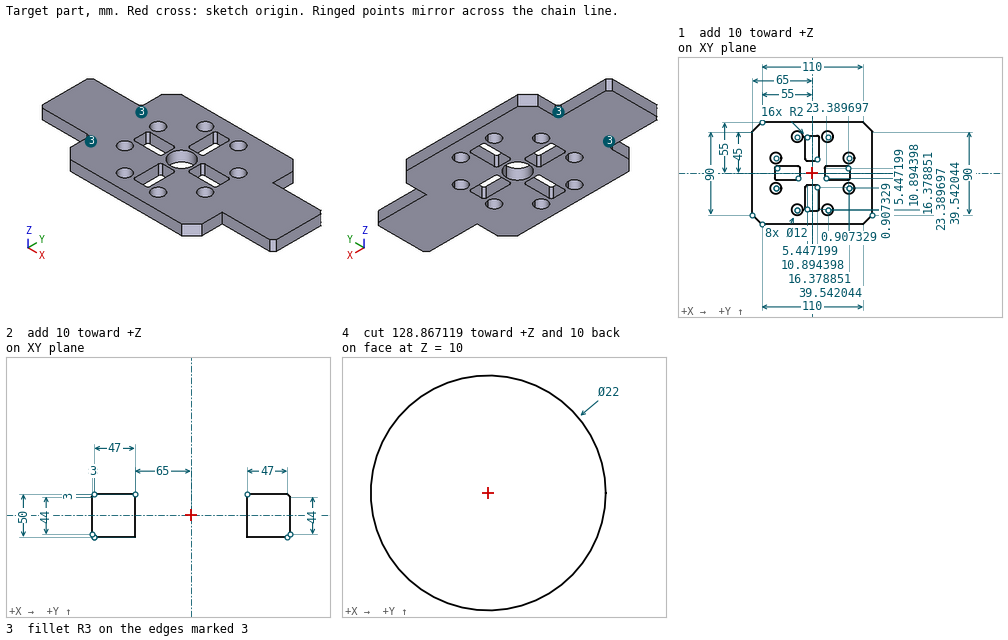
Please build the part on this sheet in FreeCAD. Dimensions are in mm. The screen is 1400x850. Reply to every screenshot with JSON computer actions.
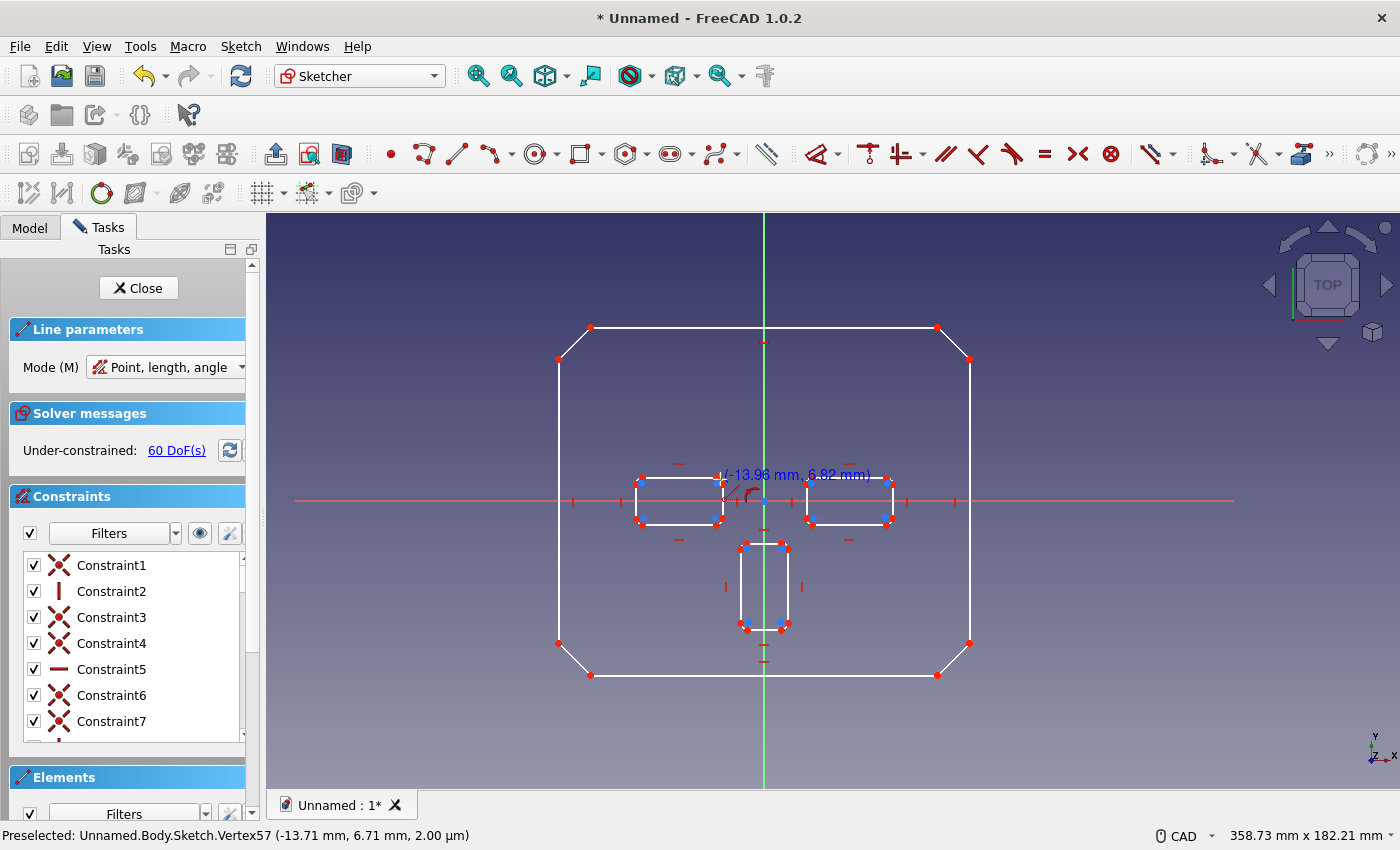
{"action": "left_click", "coordinate": [788, 379]}
{"action": "left_click", "coordinate": [788, 453]}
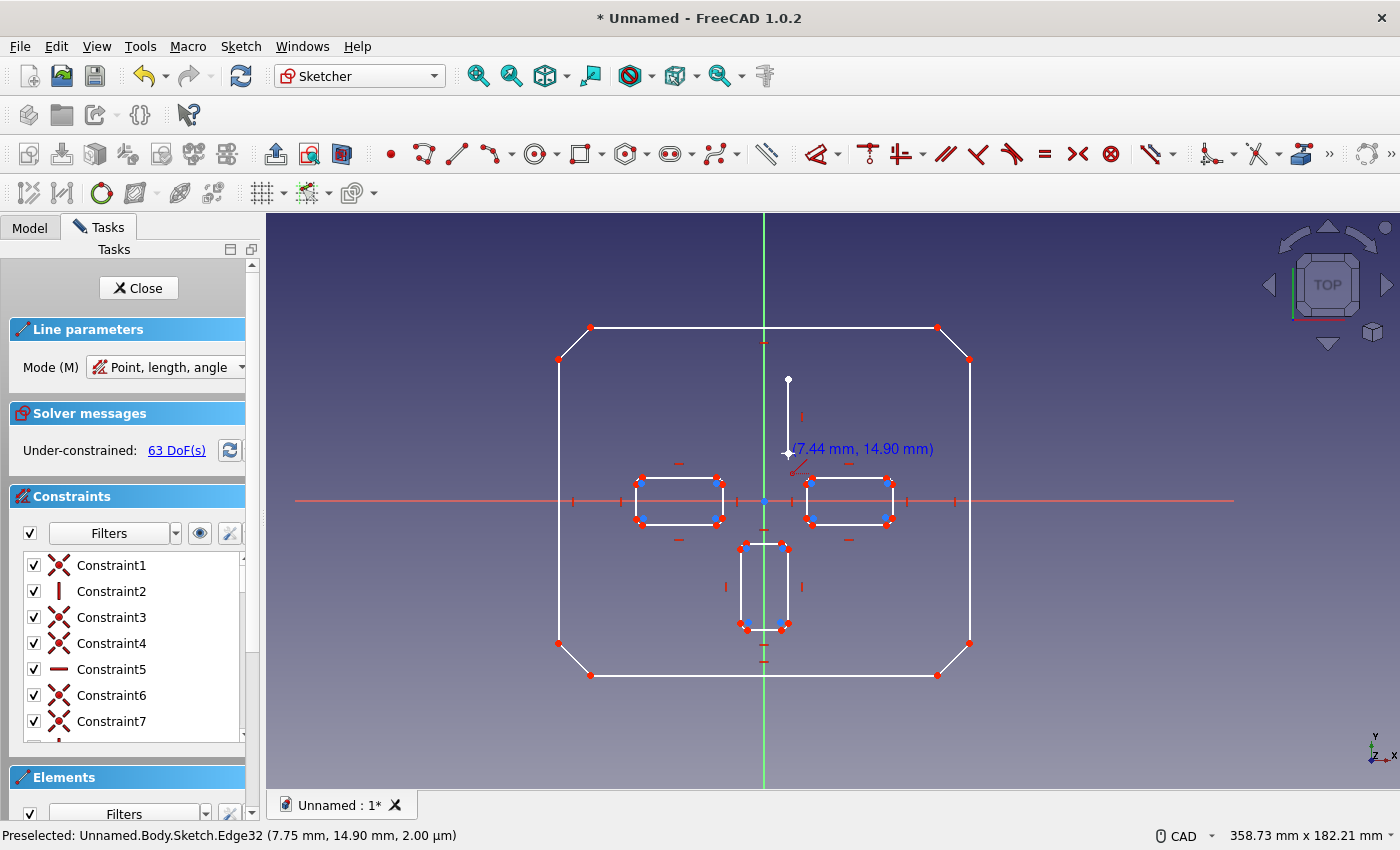
{"action": "scroll", "coordinate": [782, 459], "scroll_direction": "up", "scroll_amount": 3}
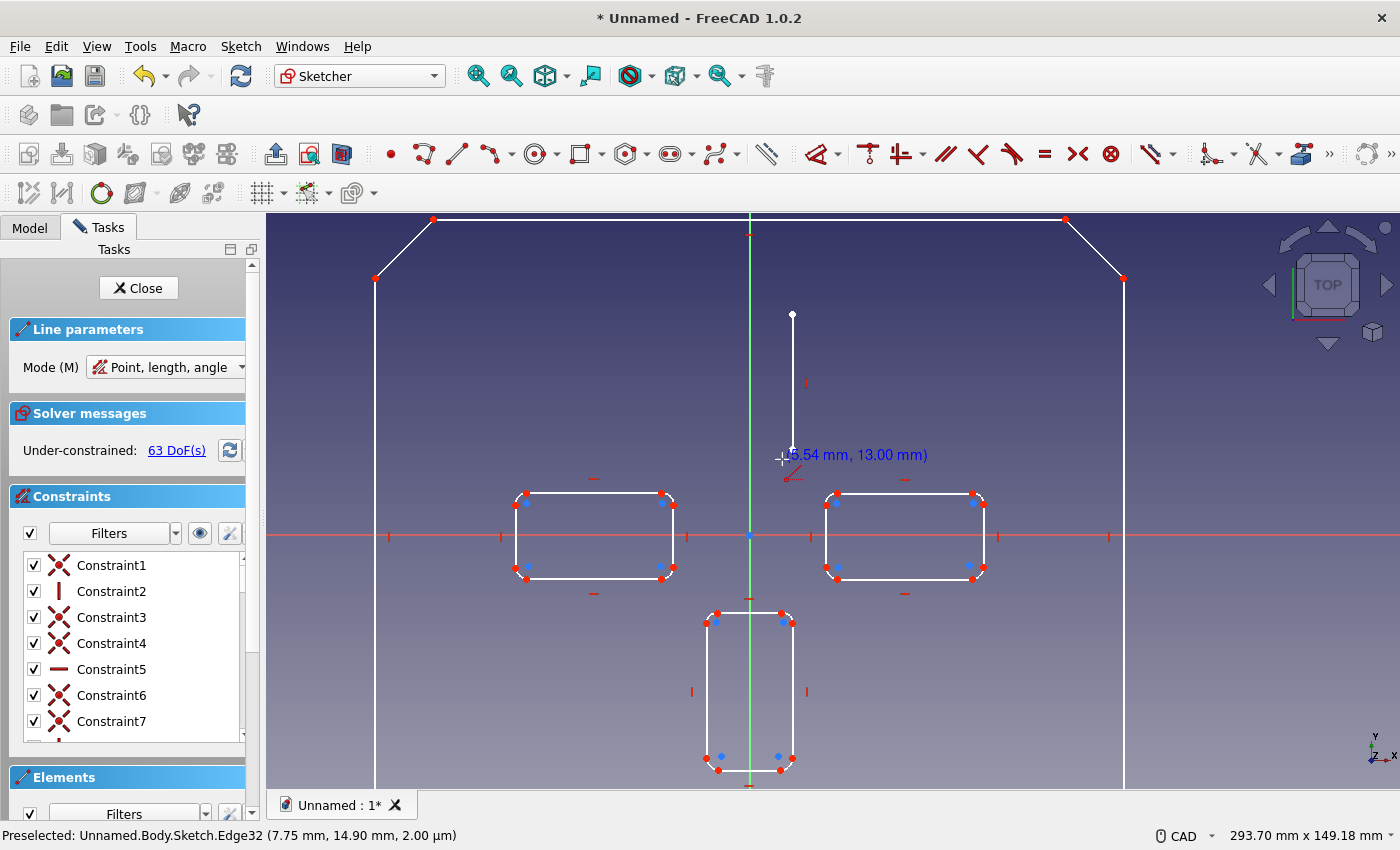
{"action": "left_click", "coordinate": [781, 459]}
{"action": "left_click", "coordinate": [718, 459]}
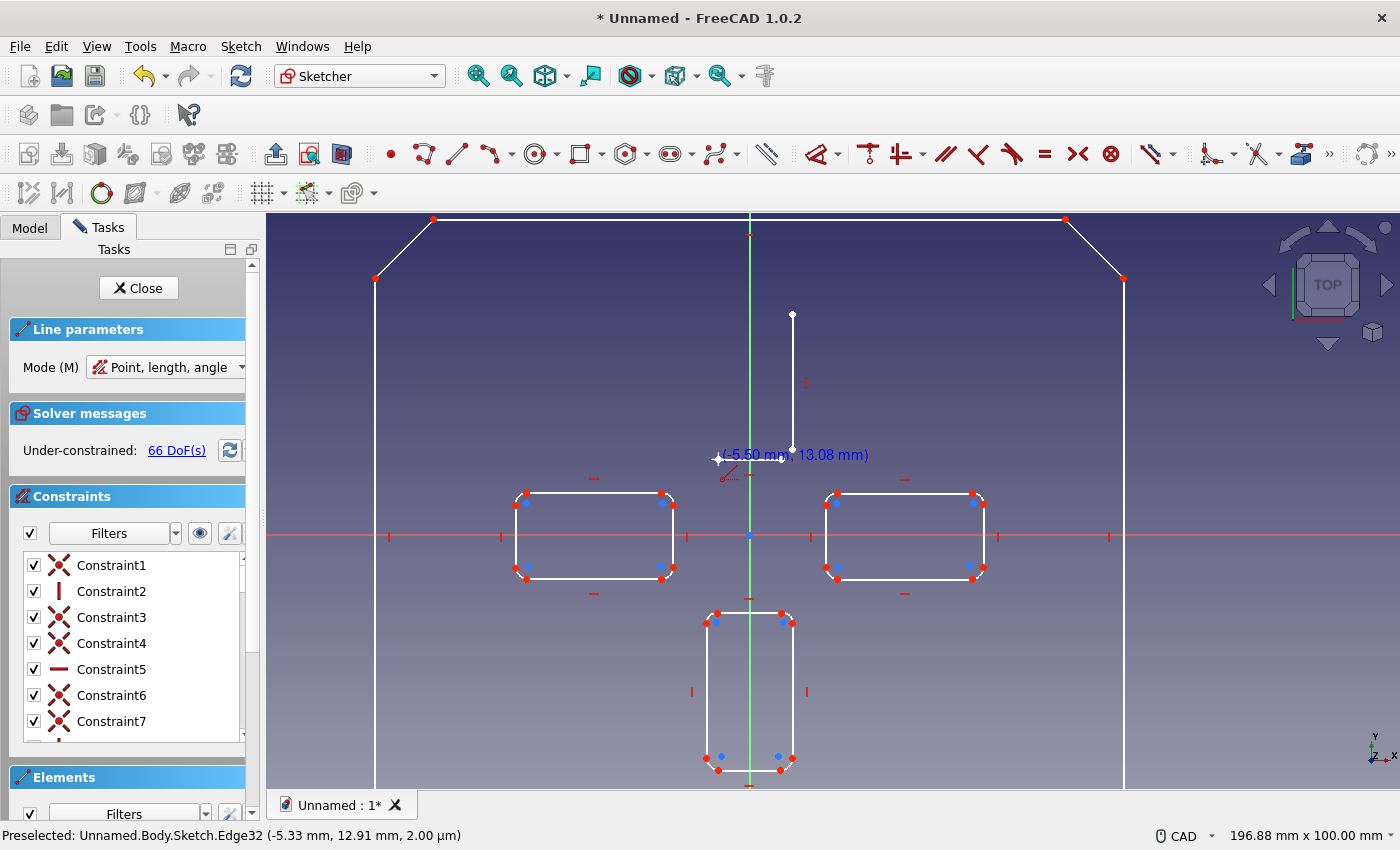
{"action": "left_click", "coordinate": [707, 448]}
{"action": "left_click", "coordinate": [707, 313]}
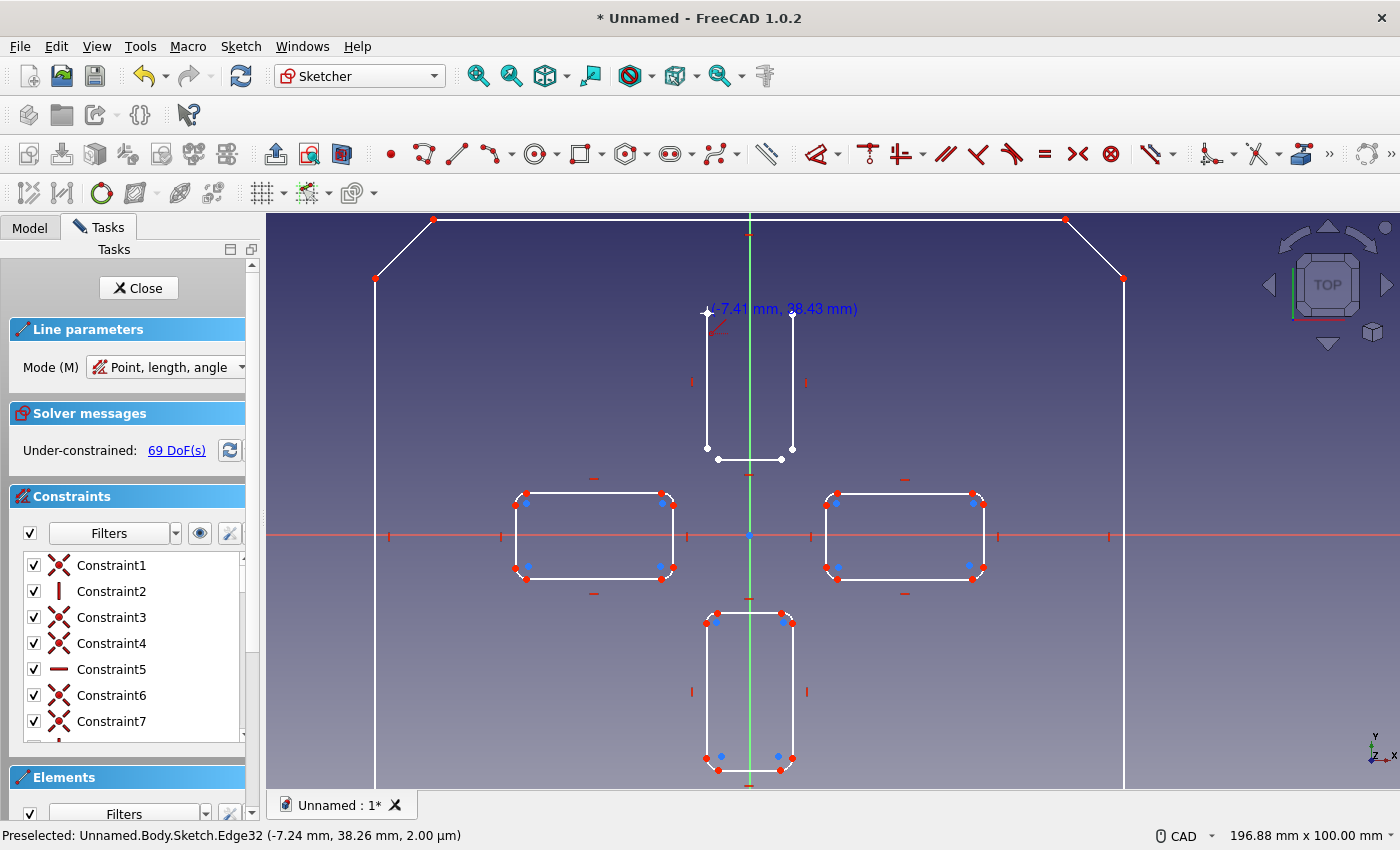
{"action": "left_click", "coordinate": [718, 301]}
{"action": "left_click", "coordinate": [781, 301]}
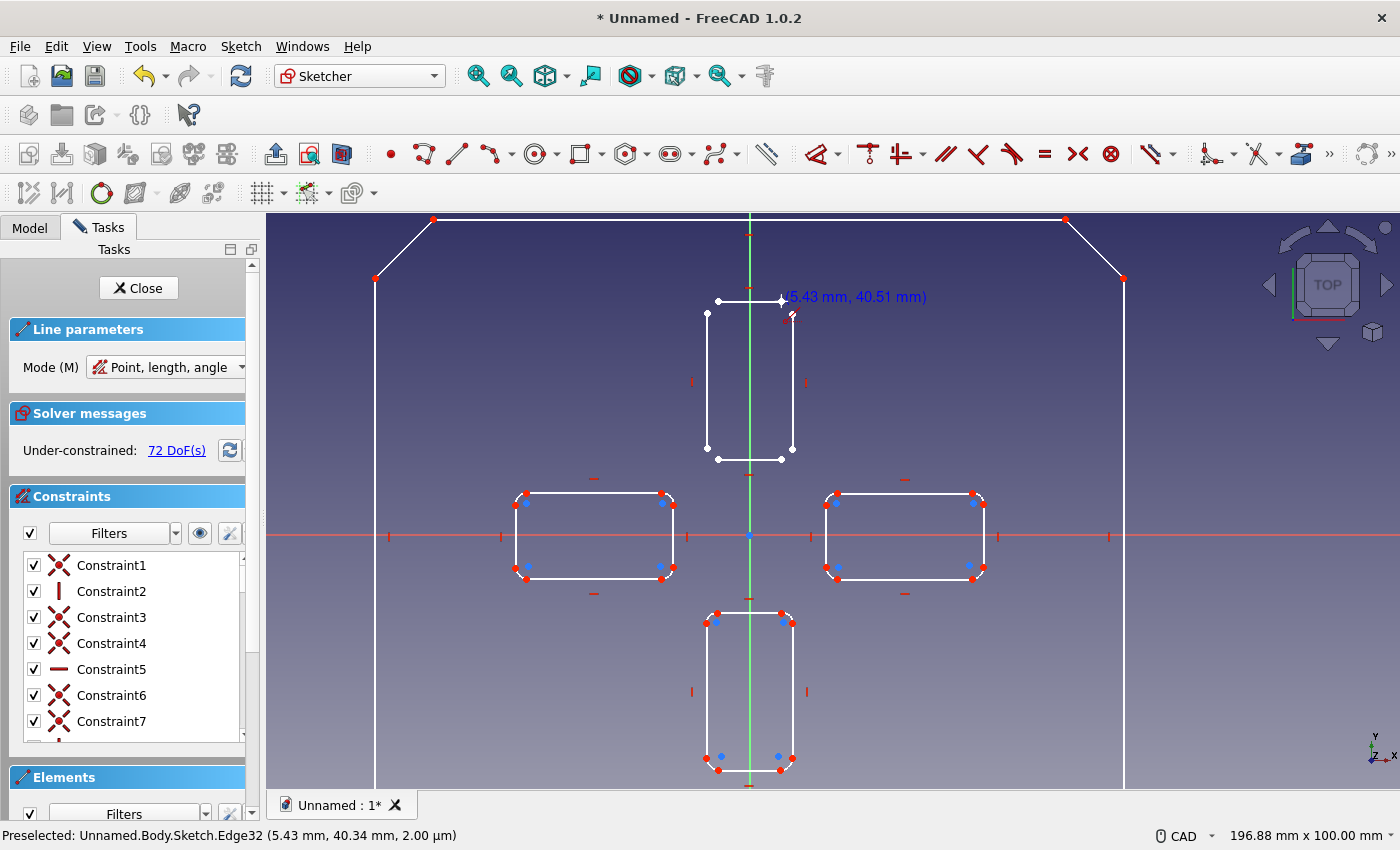
{"action": "left_click", "coordinate": [490, 154]}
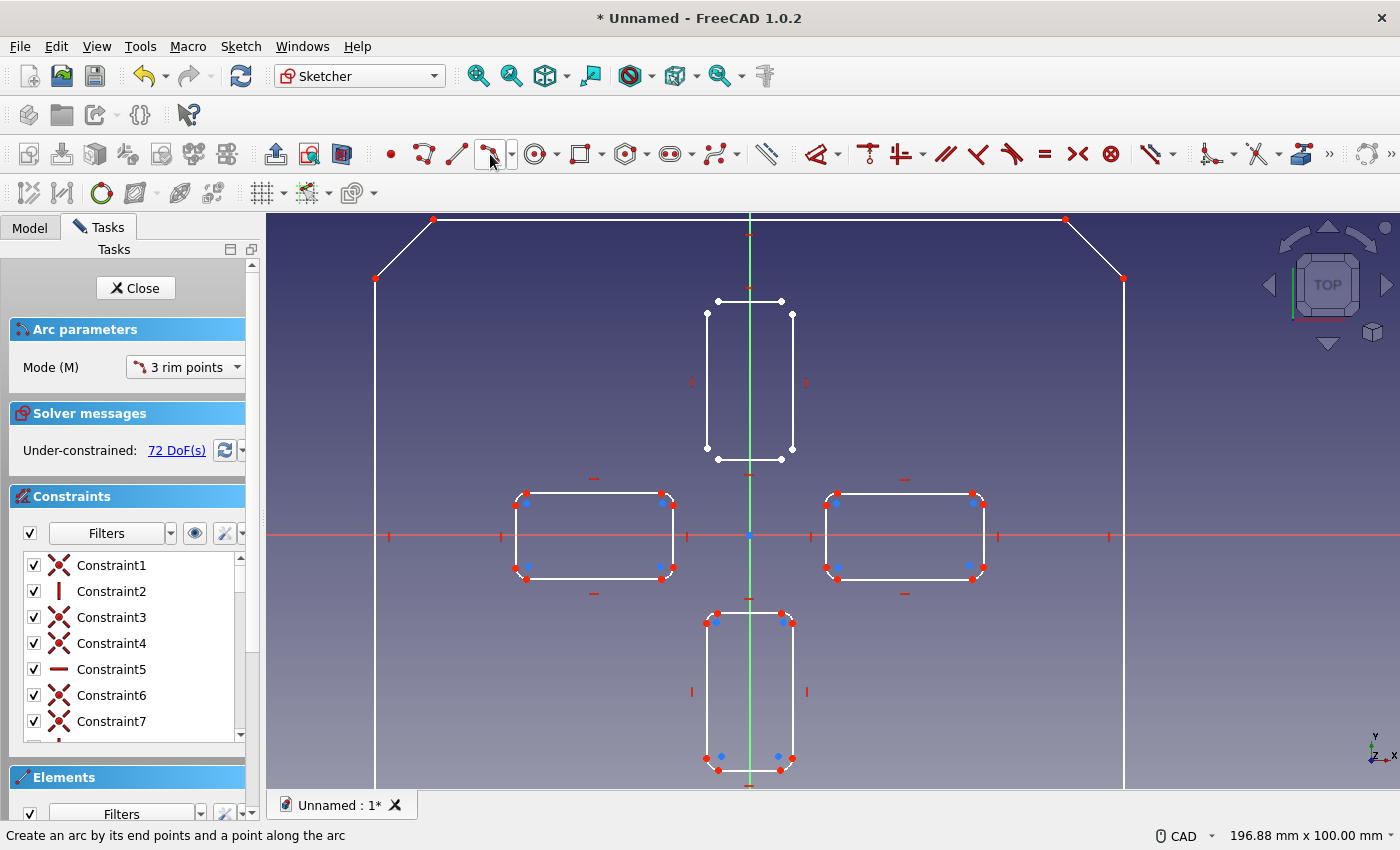
{"action": "left_click", "coordinate": [793, 450]}
{"action": "left_click", "coordinate": [781, 460]}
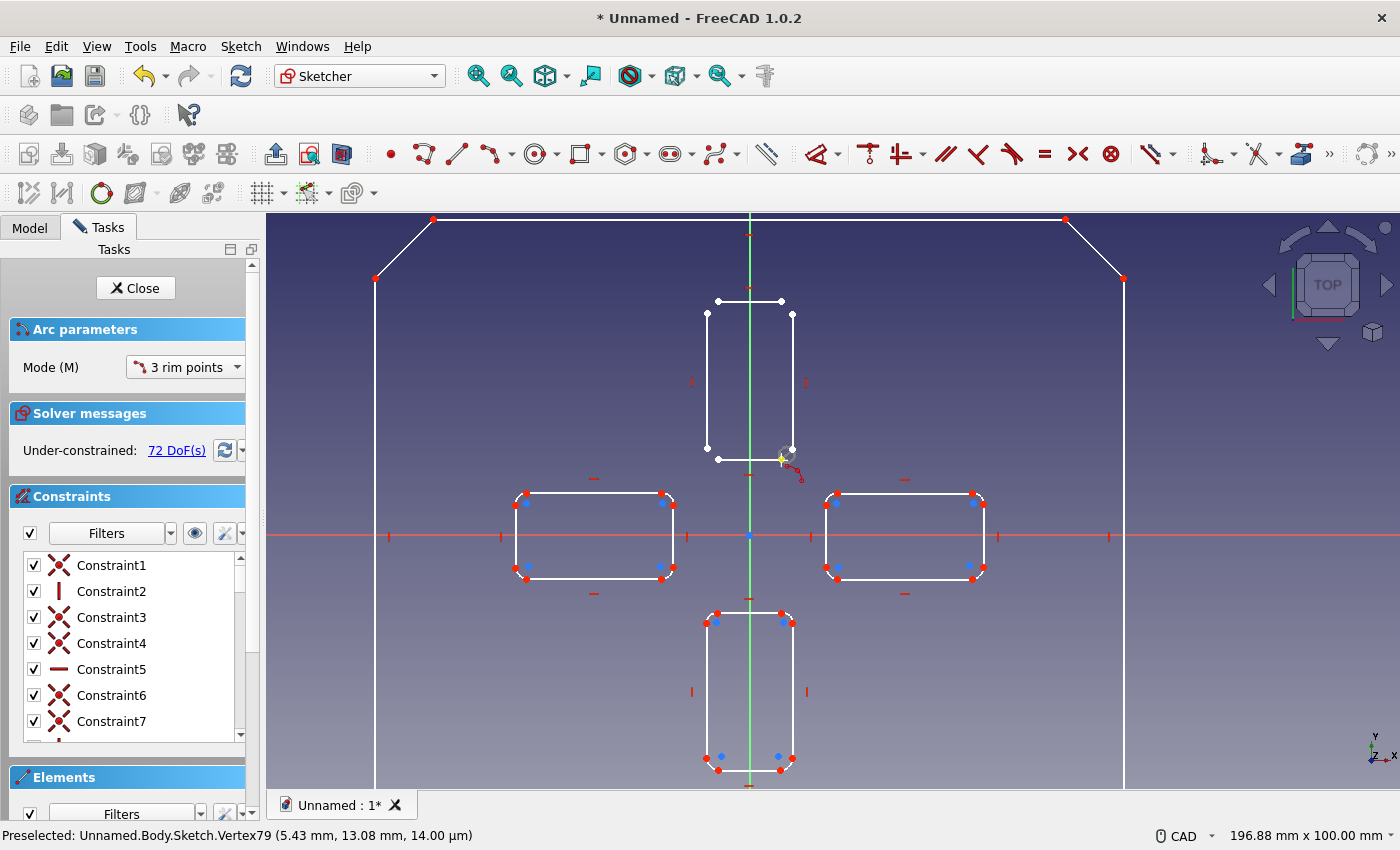
{"action": "scroll", "coordinate": [789, 456], "scroll_direction": "up", "scroll_amount": 8}